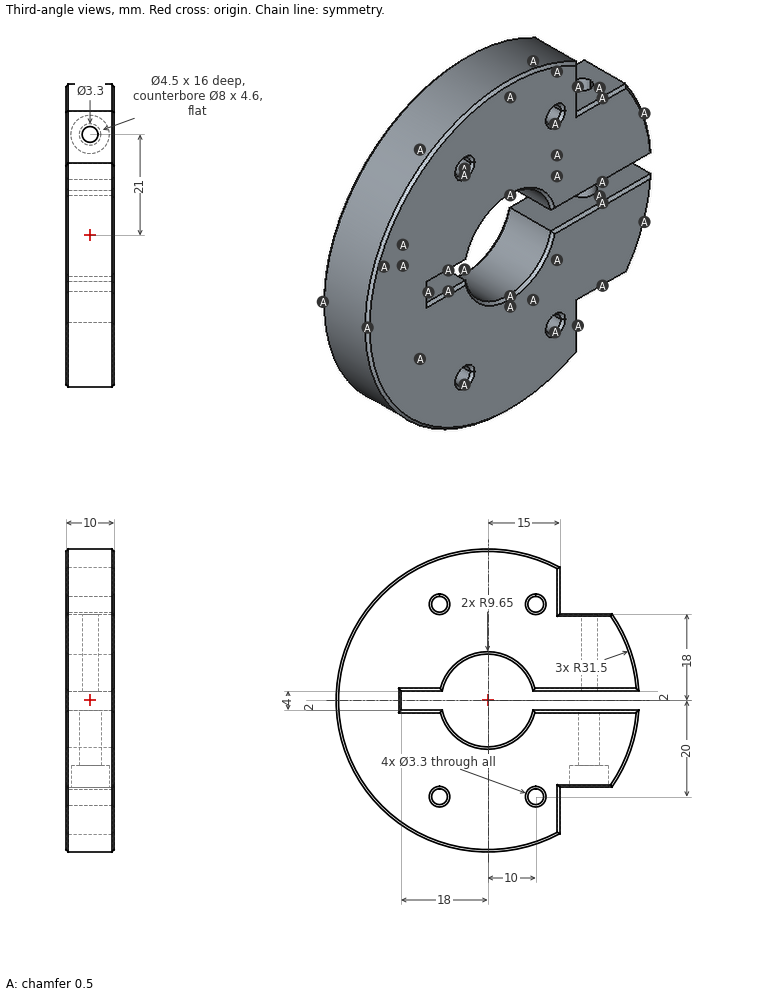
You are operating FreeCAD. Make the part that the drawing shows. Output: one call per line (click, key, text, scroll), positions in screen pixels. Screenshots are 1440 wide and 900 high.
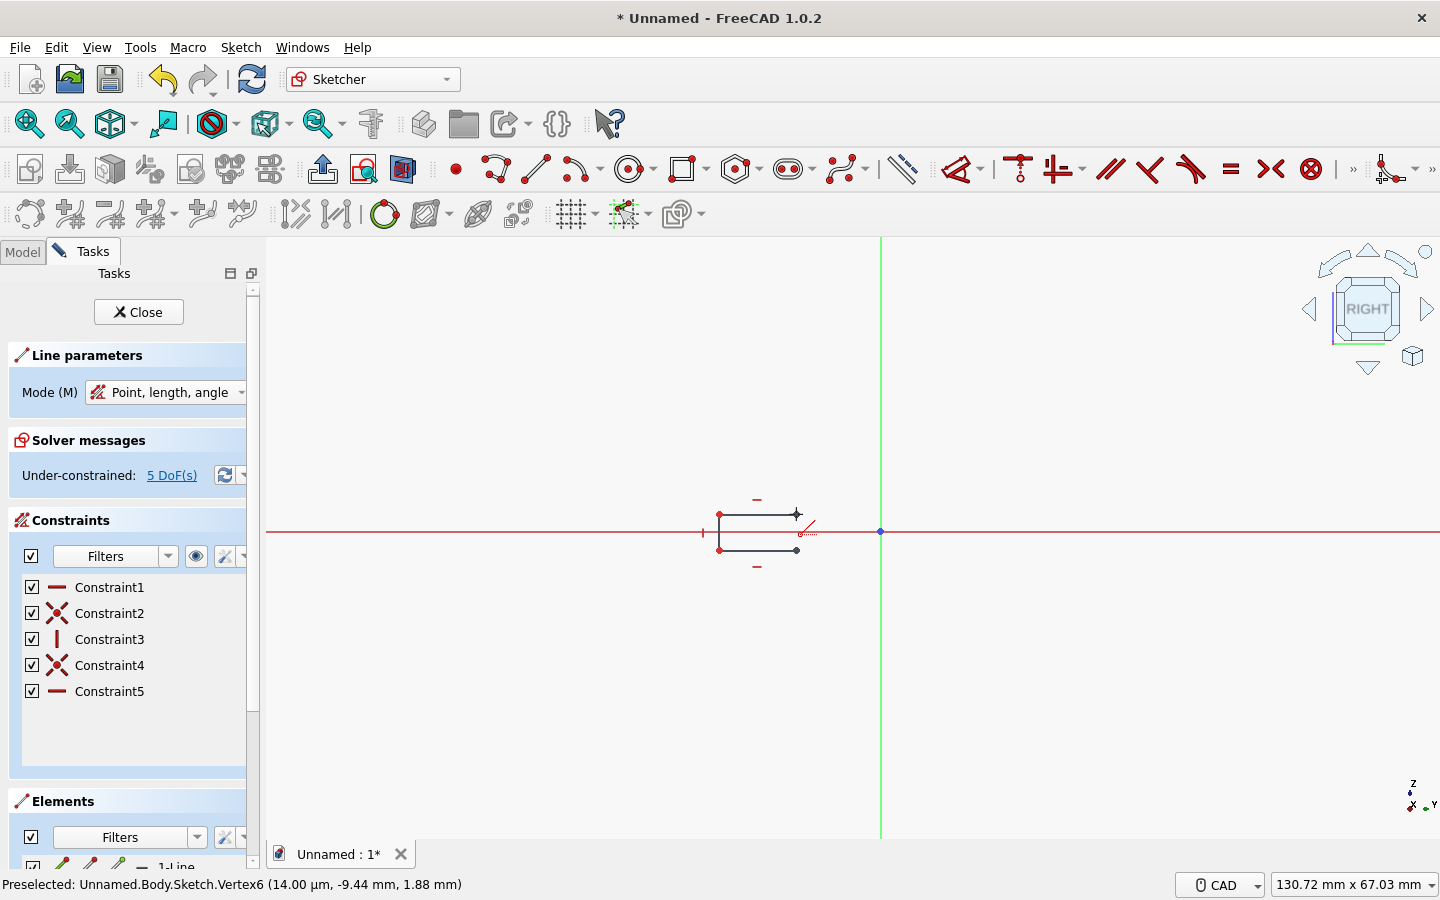
click(966, 514)
click(1163, 514)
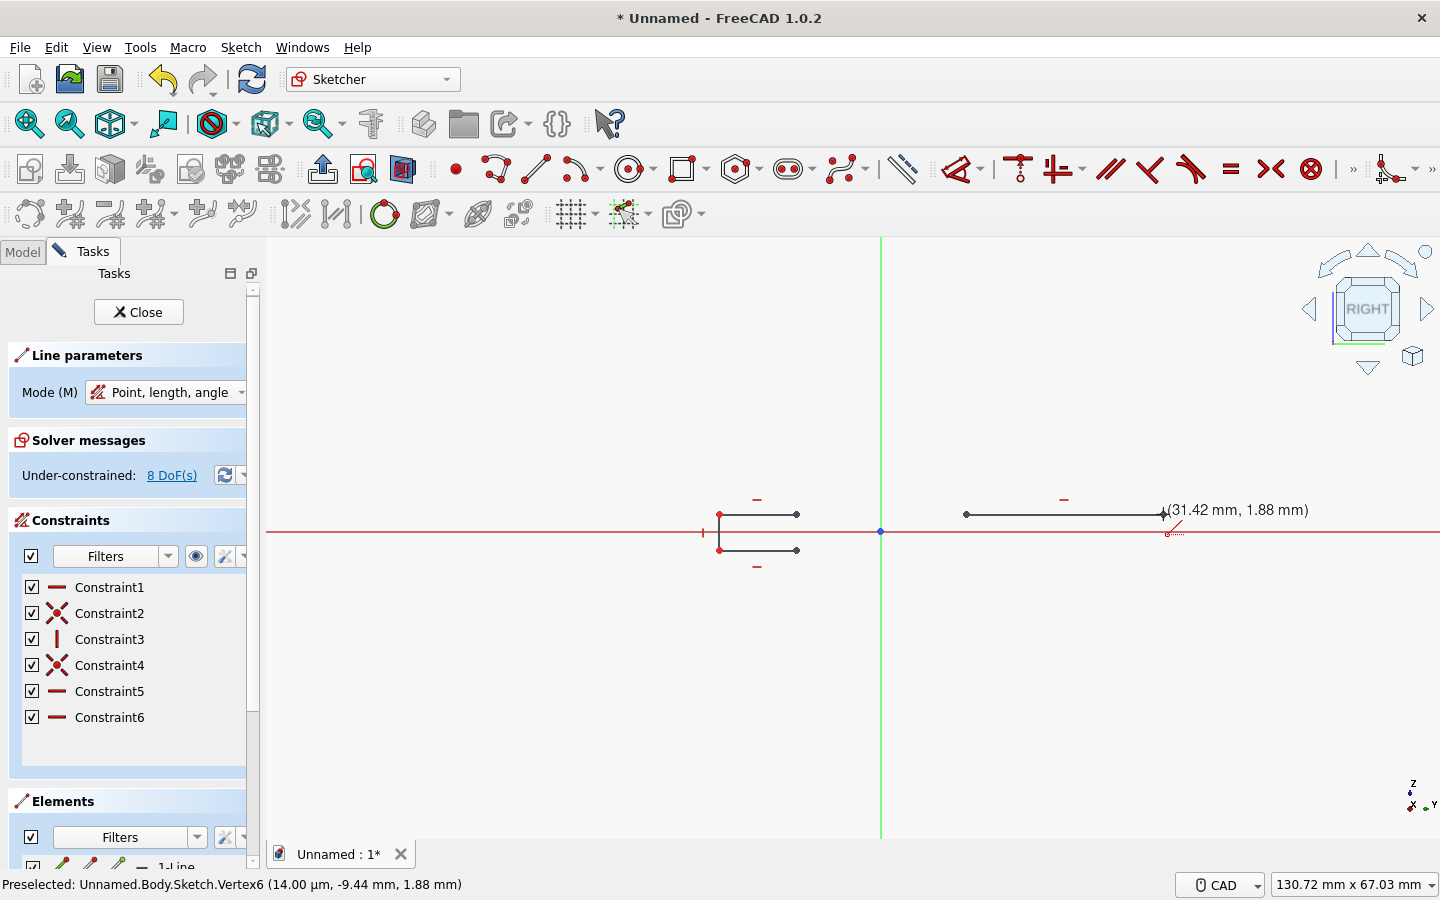
key(g)
key(m)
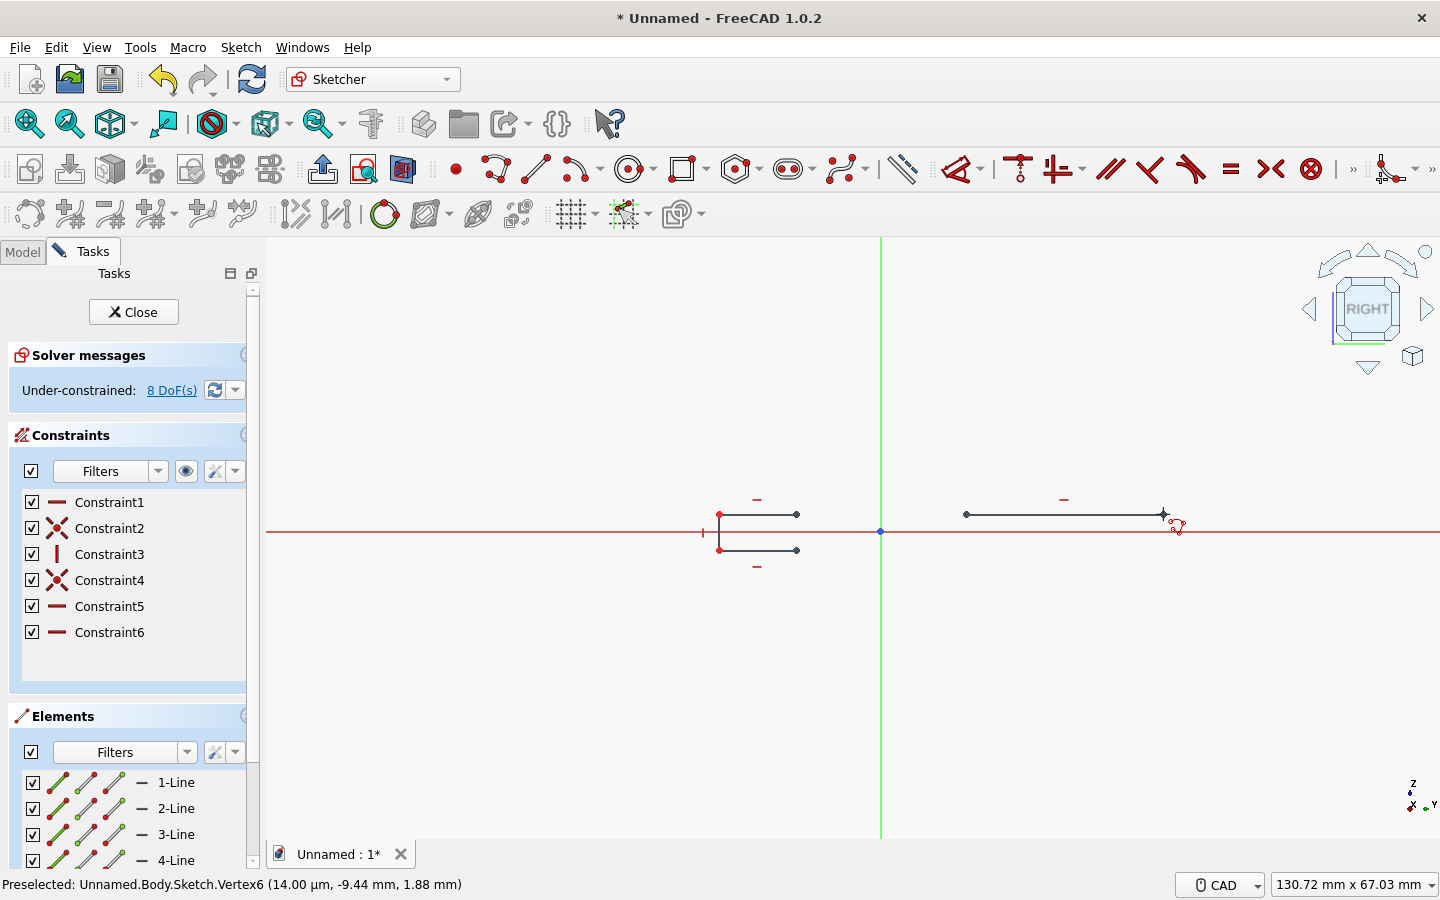
click(1113, 370)
click(1016, 370)
click(1016, 283)
right_click(1016, 283)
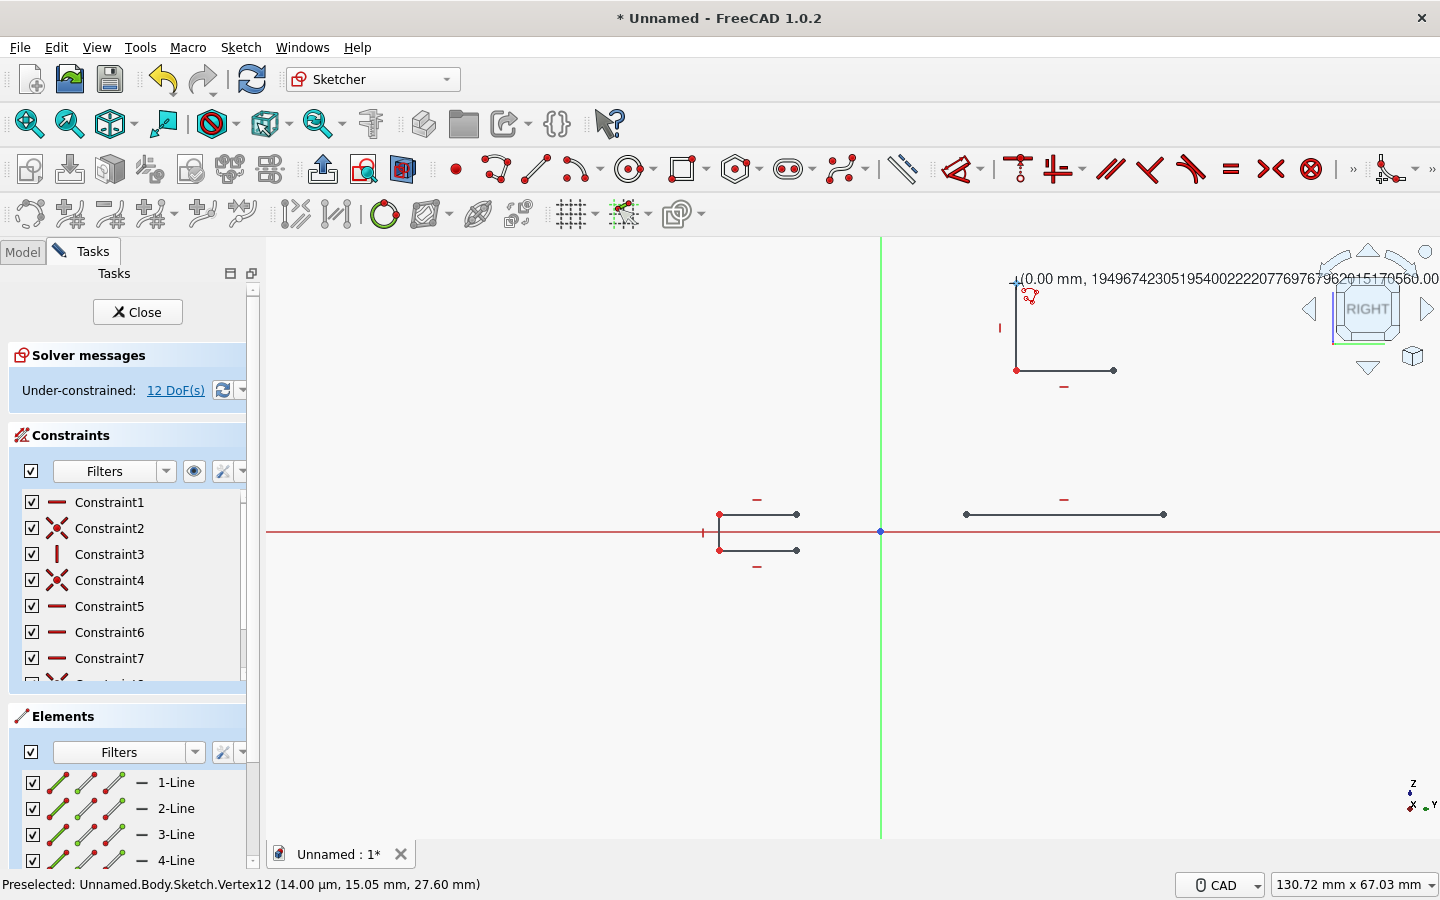
click(1016, 781)
click(1016, 693)
click(1113, 693)
right_click(1113, 693)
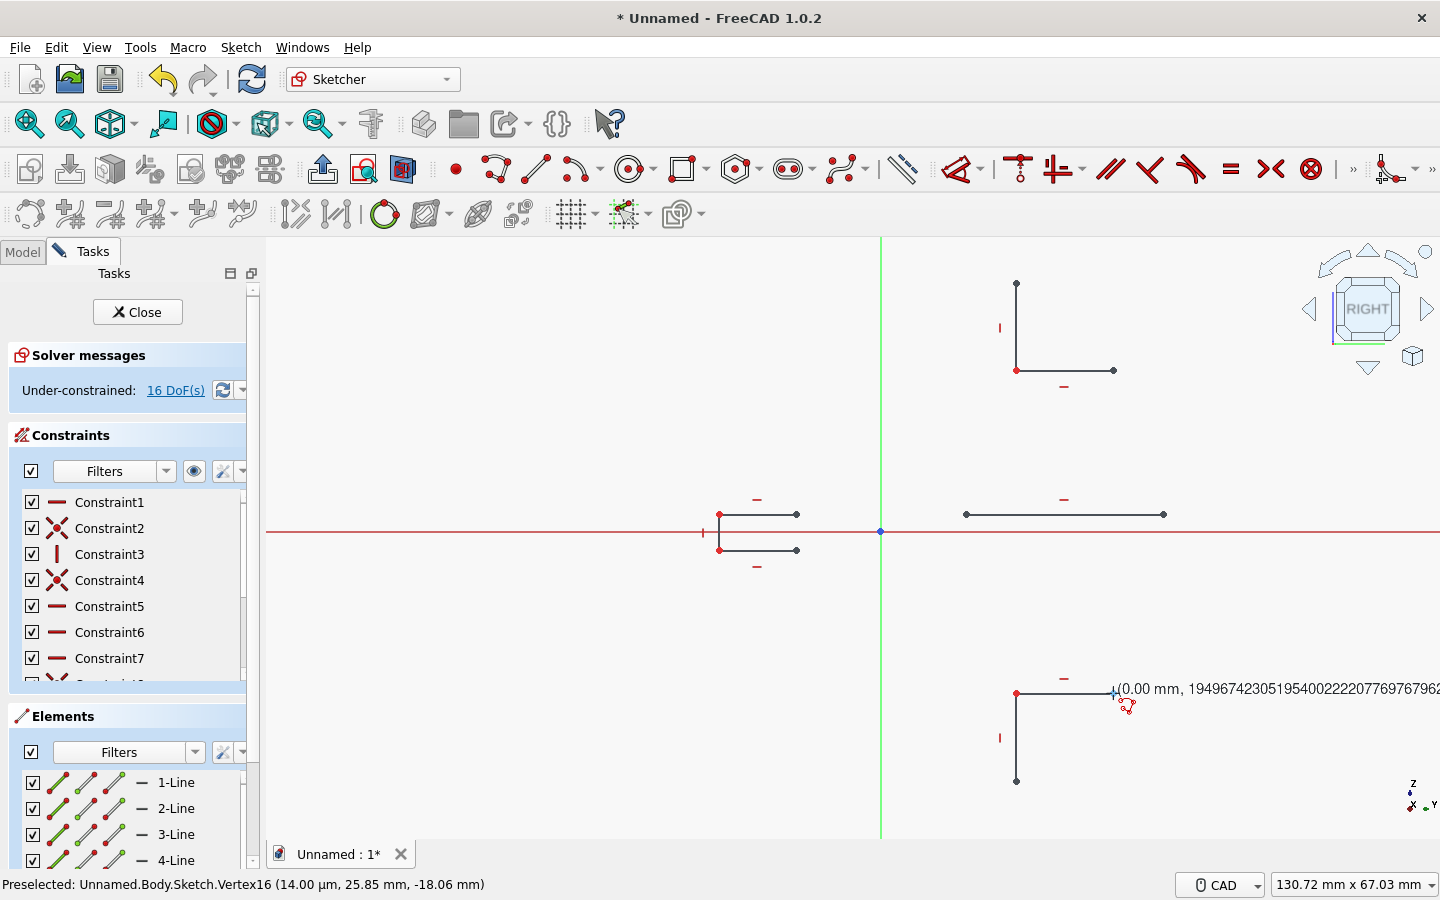
key(g)
key(l)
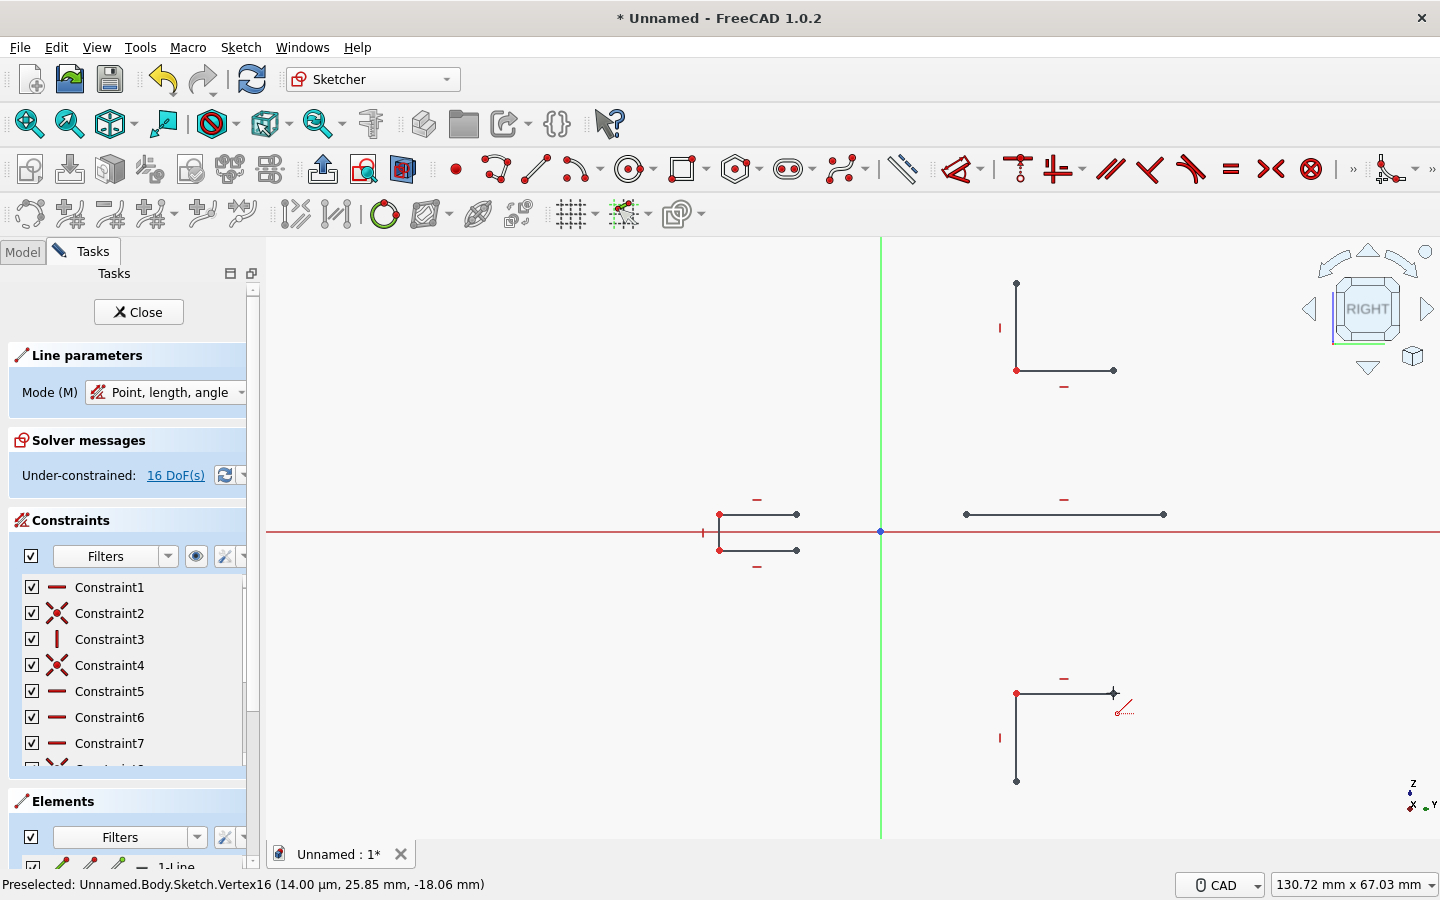
click(1163, 550)
click(966, 550)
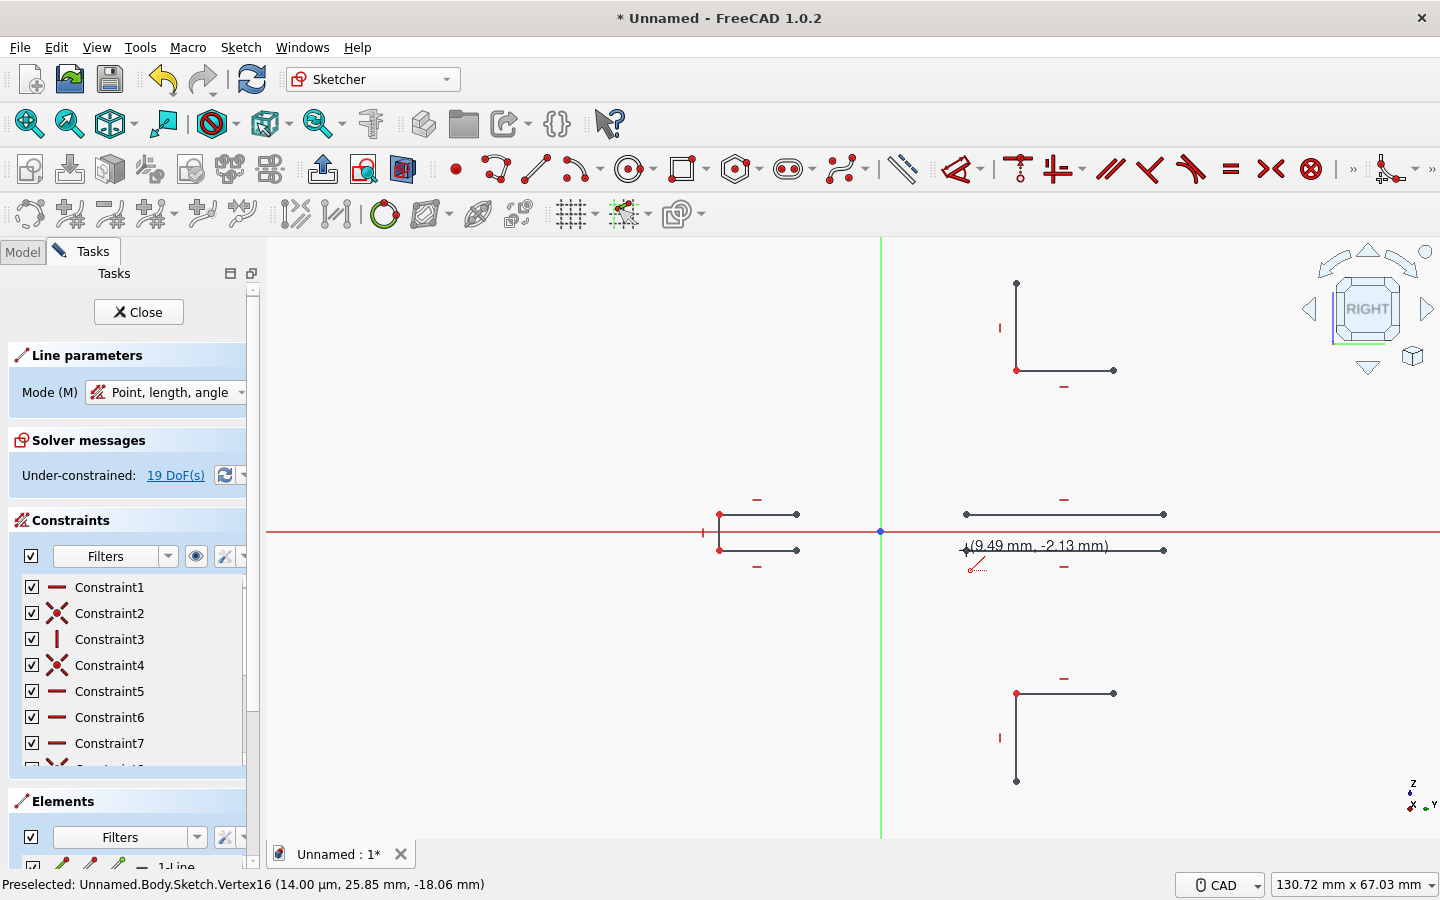
key(g)
key(3)
key(a)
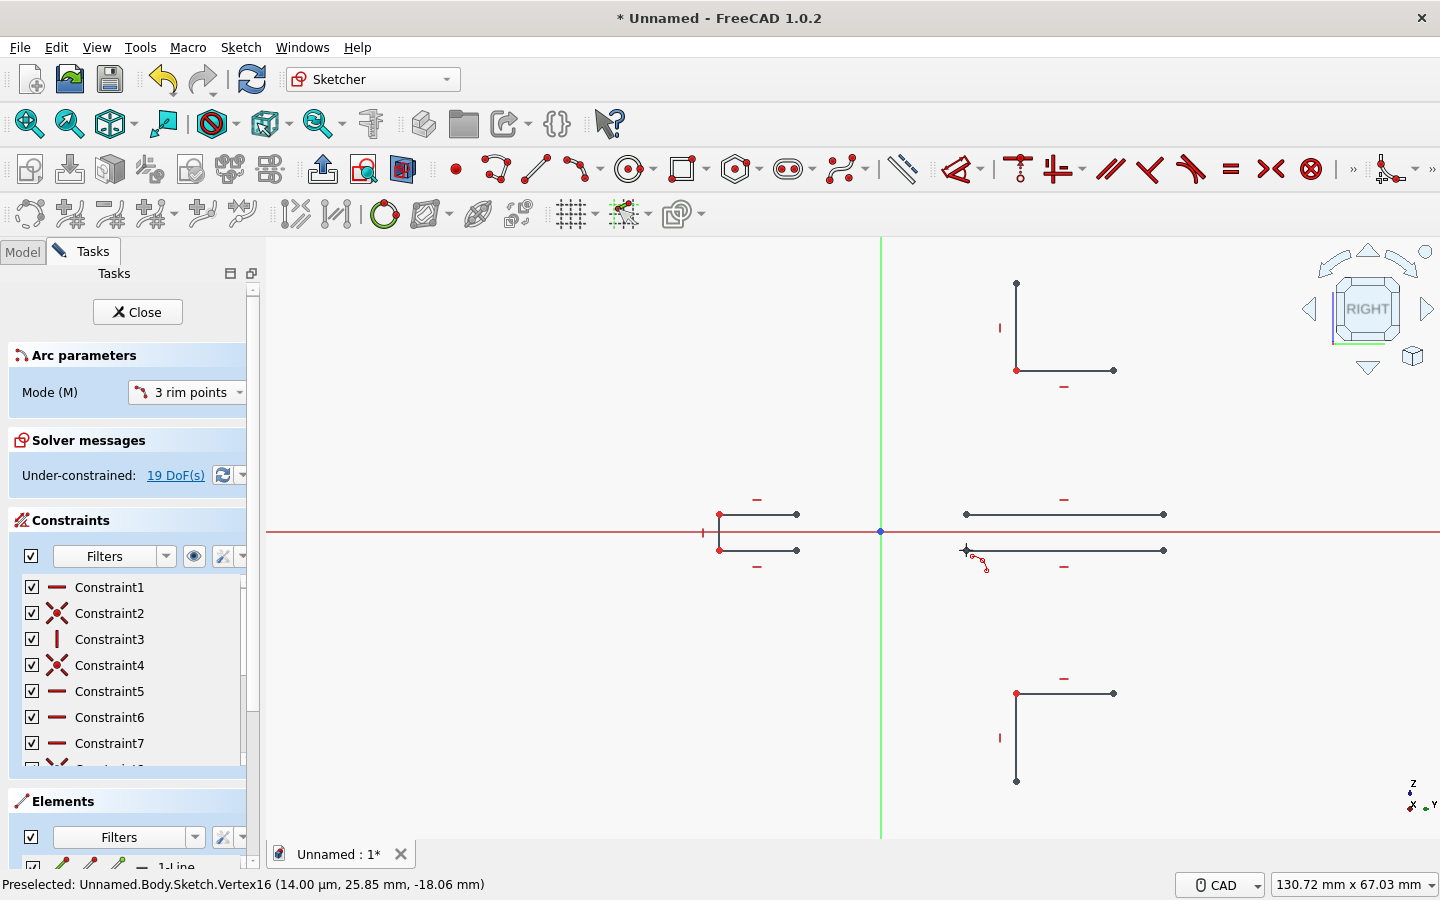
click(796, 515)
click(966, 515)
click(904, 448)